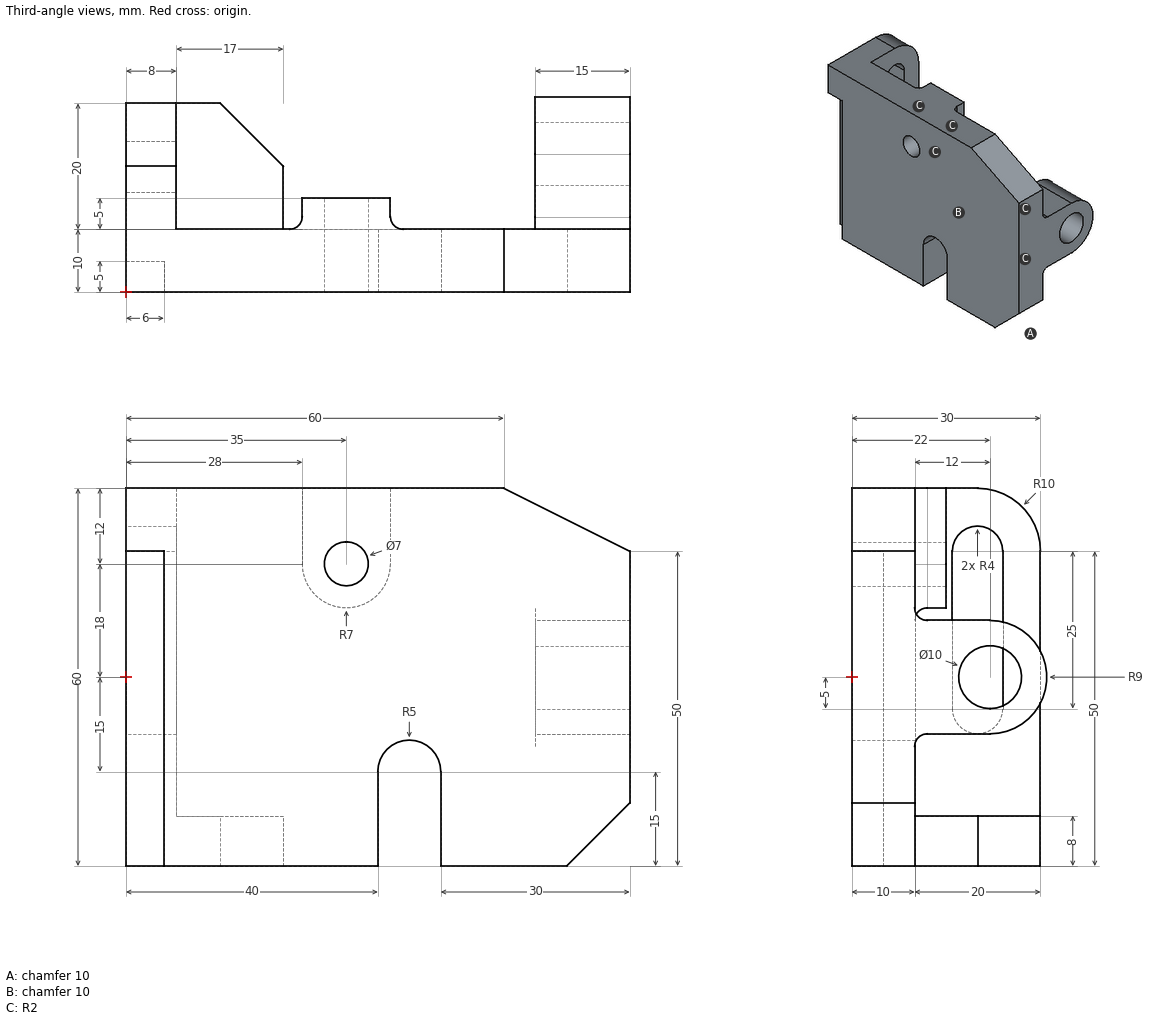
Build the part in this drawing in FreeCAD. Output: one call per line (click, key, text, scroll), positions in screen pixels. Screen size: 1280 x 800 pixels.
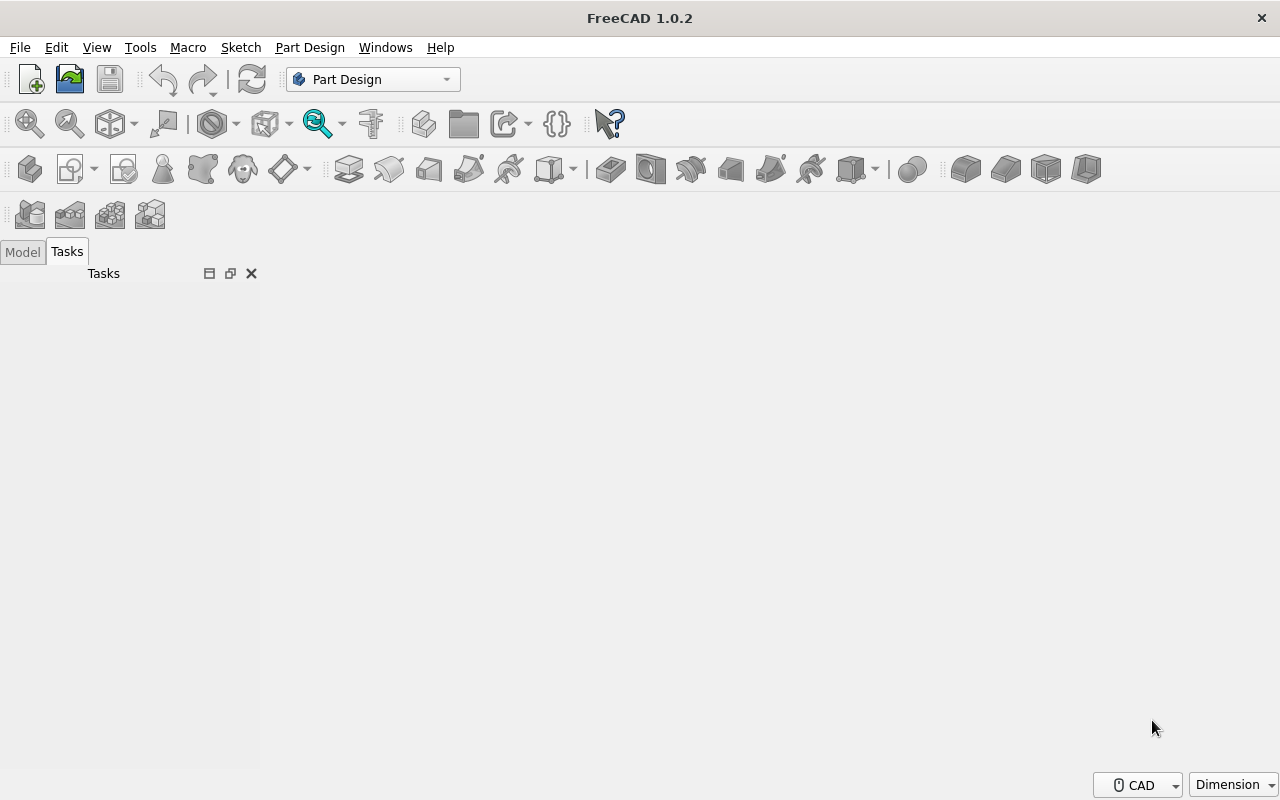
click(30, 80)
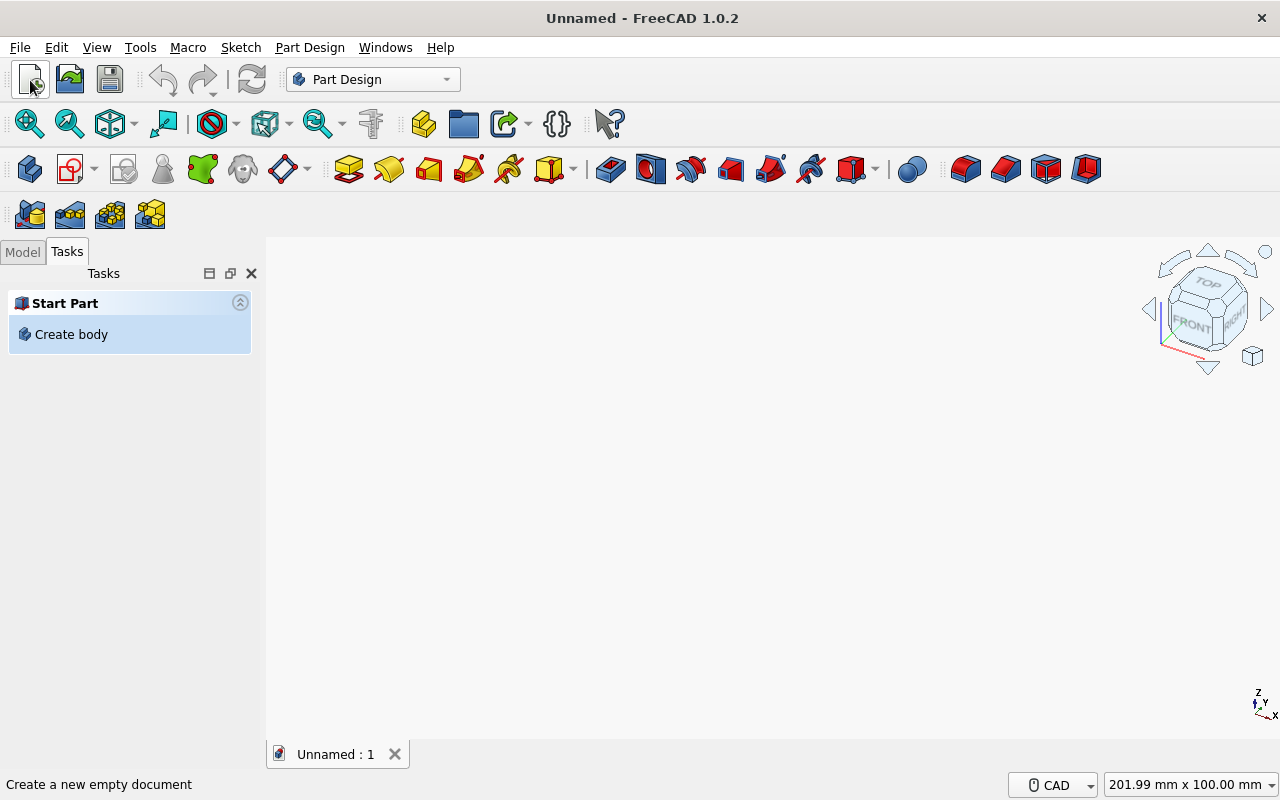
click(70, 170)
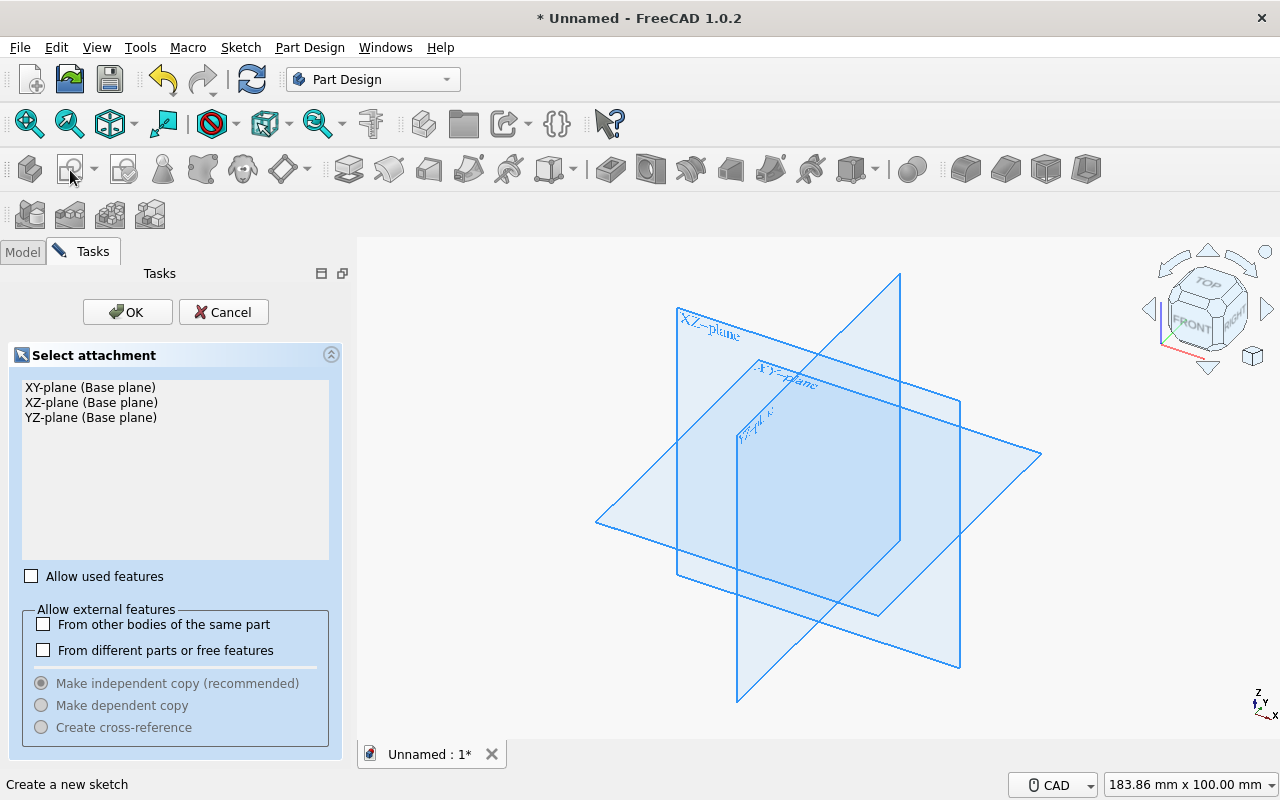
click(82, 402)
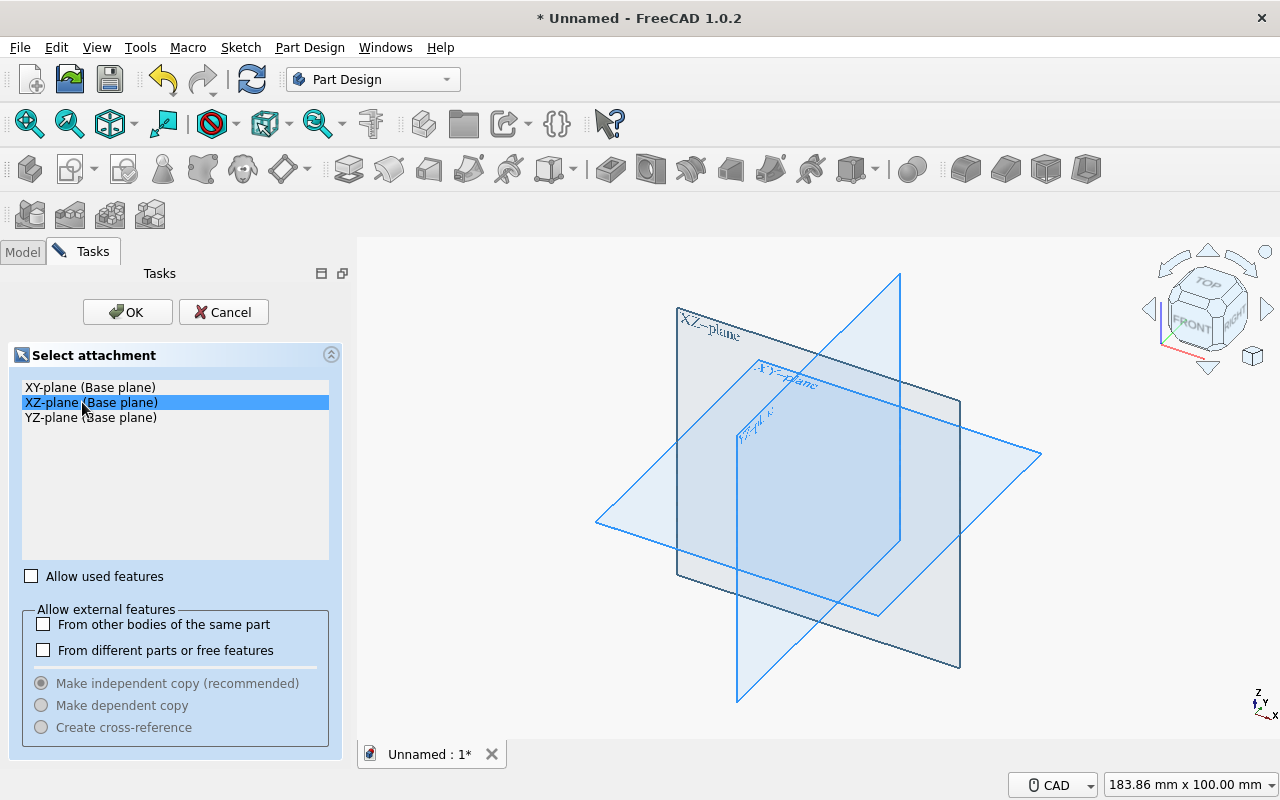
click(128, 312)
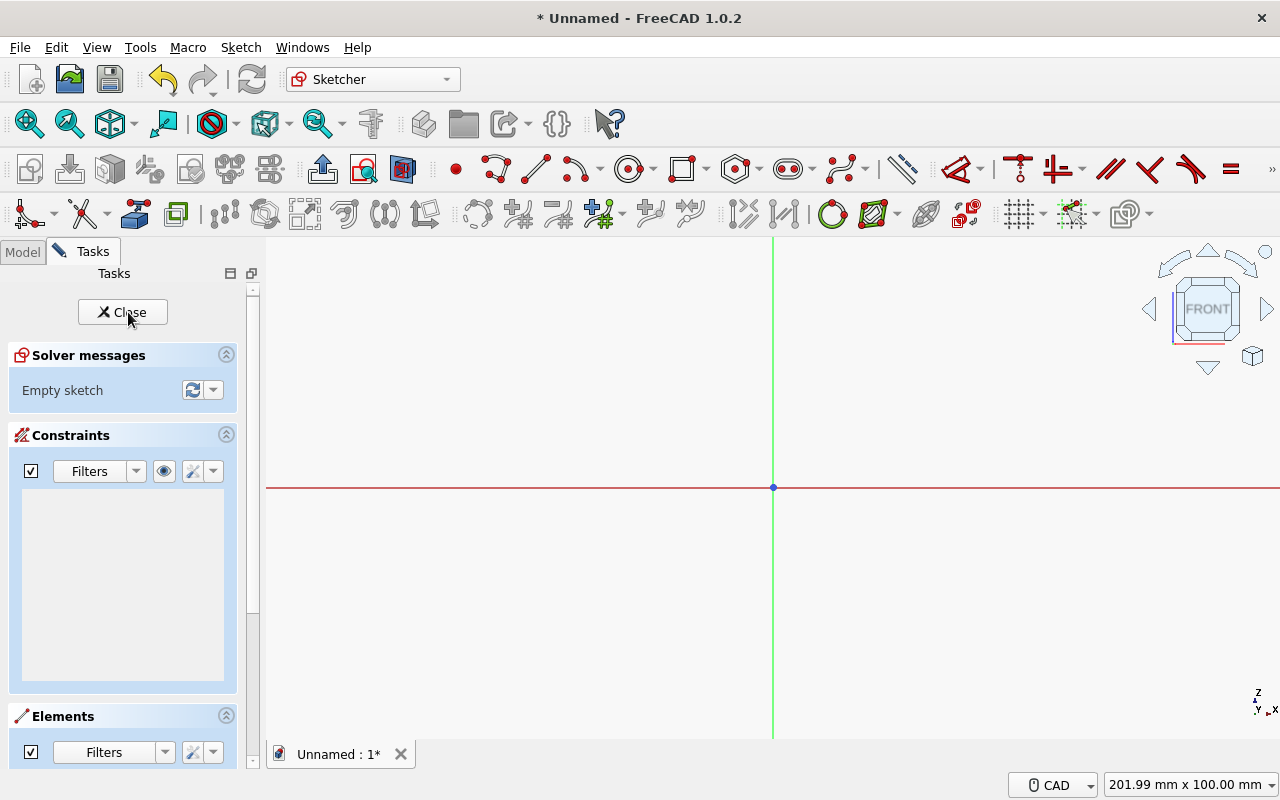
scroll(294, 488, down, 1)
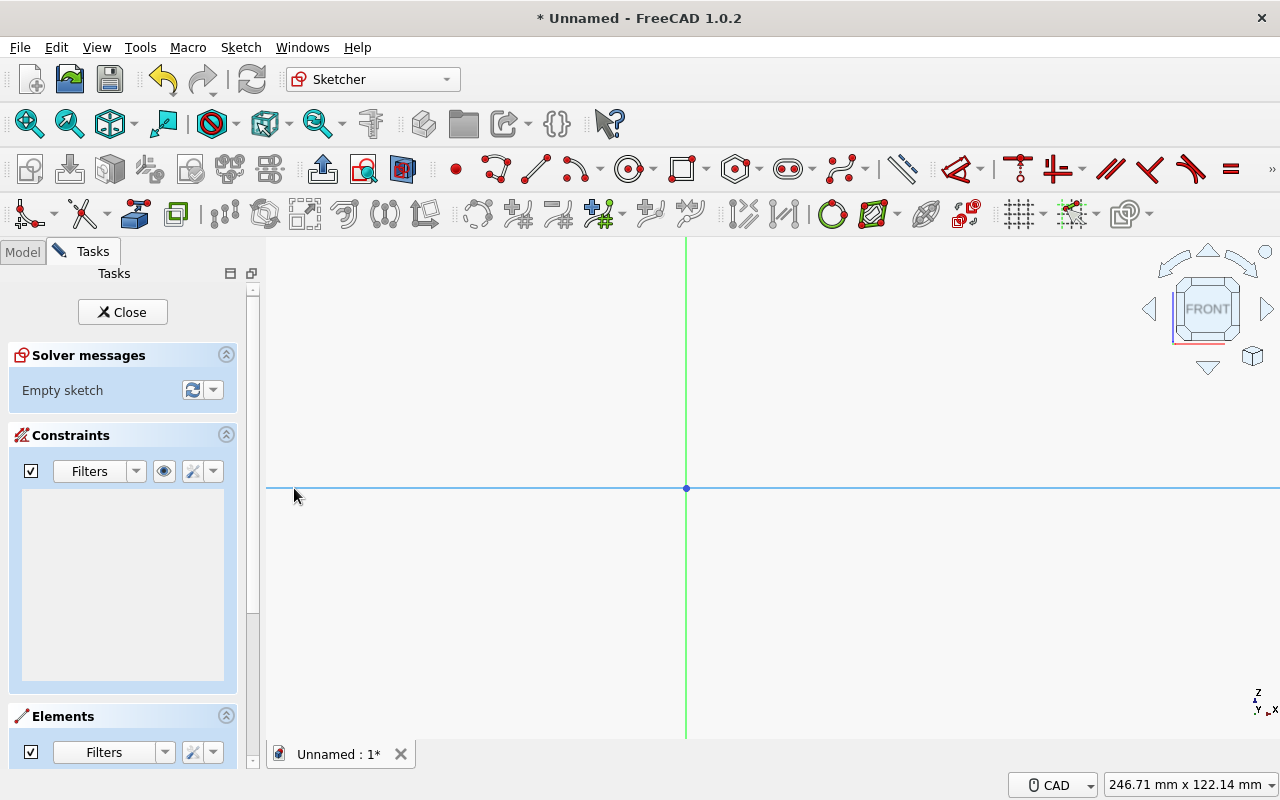
click(496, 170)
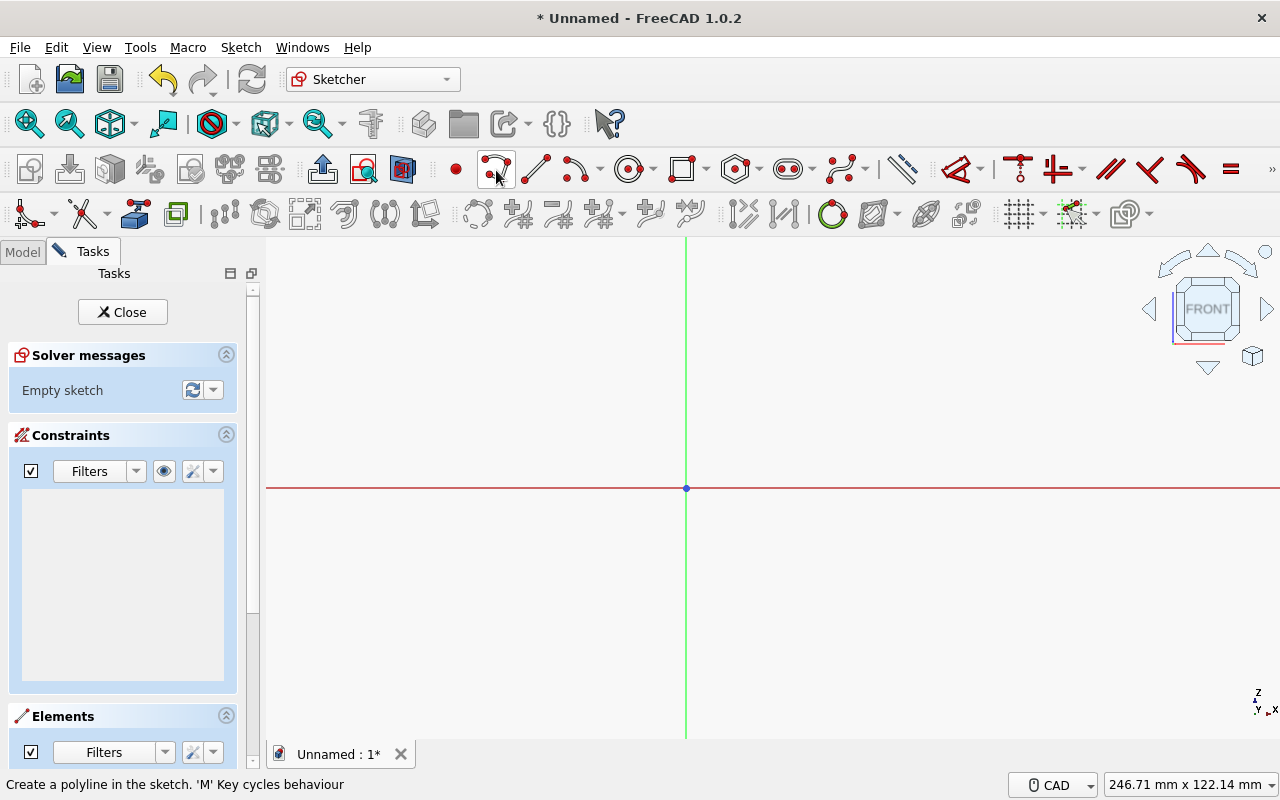
click(851, 550)
click(851, 611)
click(686, 611)
click(695, 365)
click(933, 365)
click(1015, 406)
click(1015, 611)
click(892, 611)
click(892, 550)
right_click(892, 550)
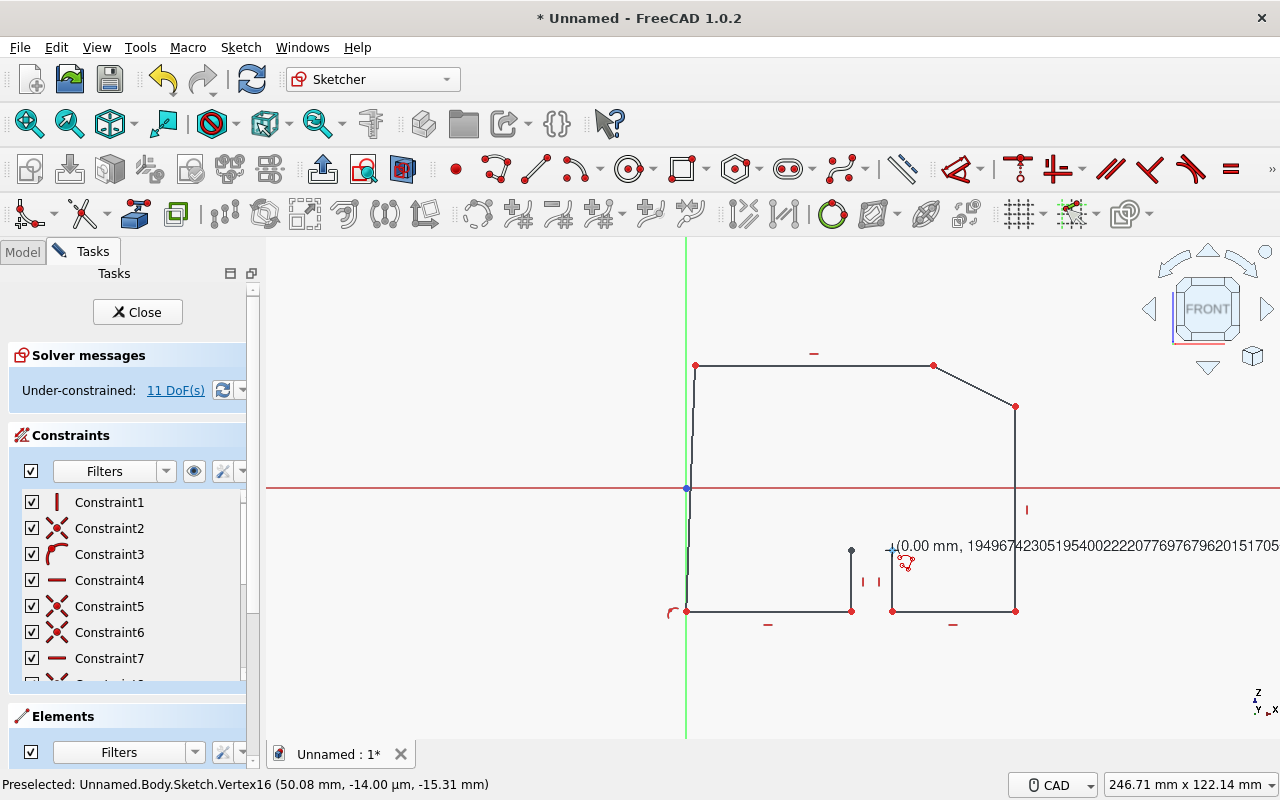
key(g)
key(3)
key(a)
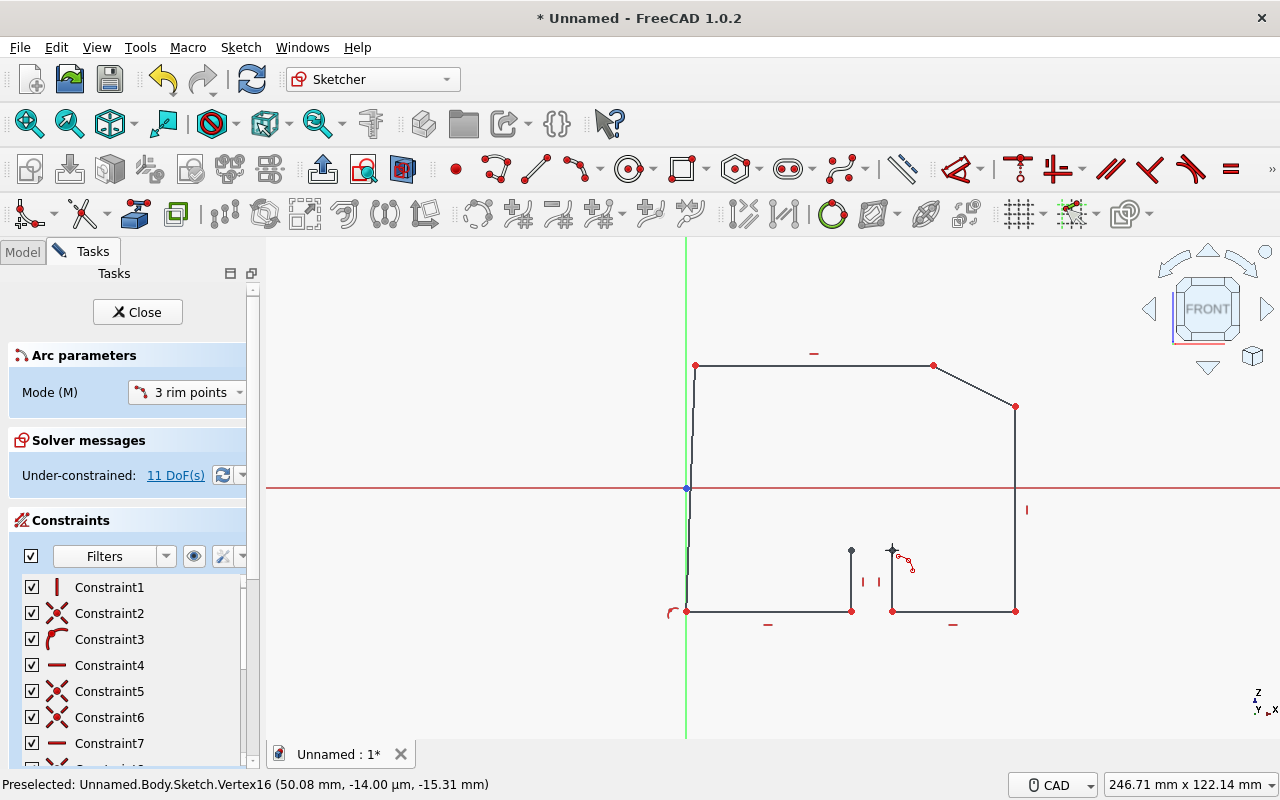
click(892, 551)
click(851, 551)
click(871, 529)
key(Escape)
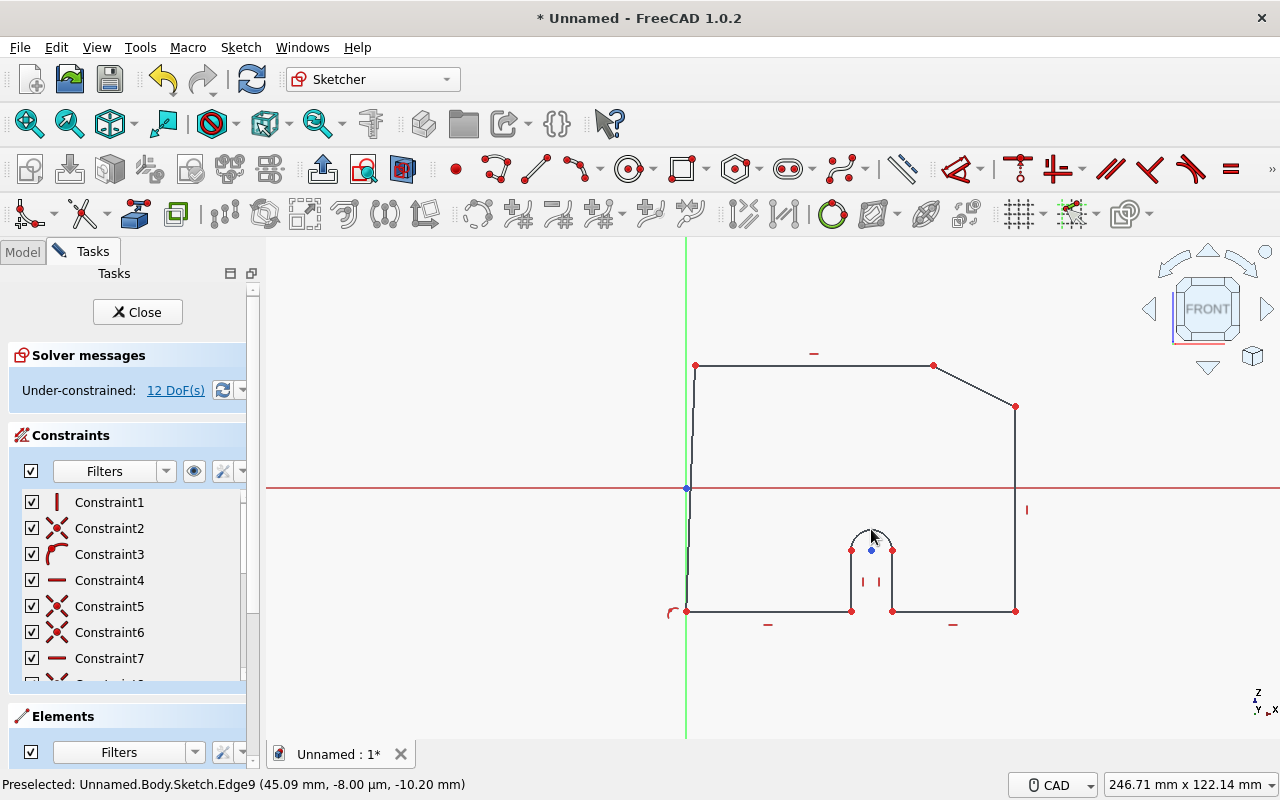
click(851, 569)